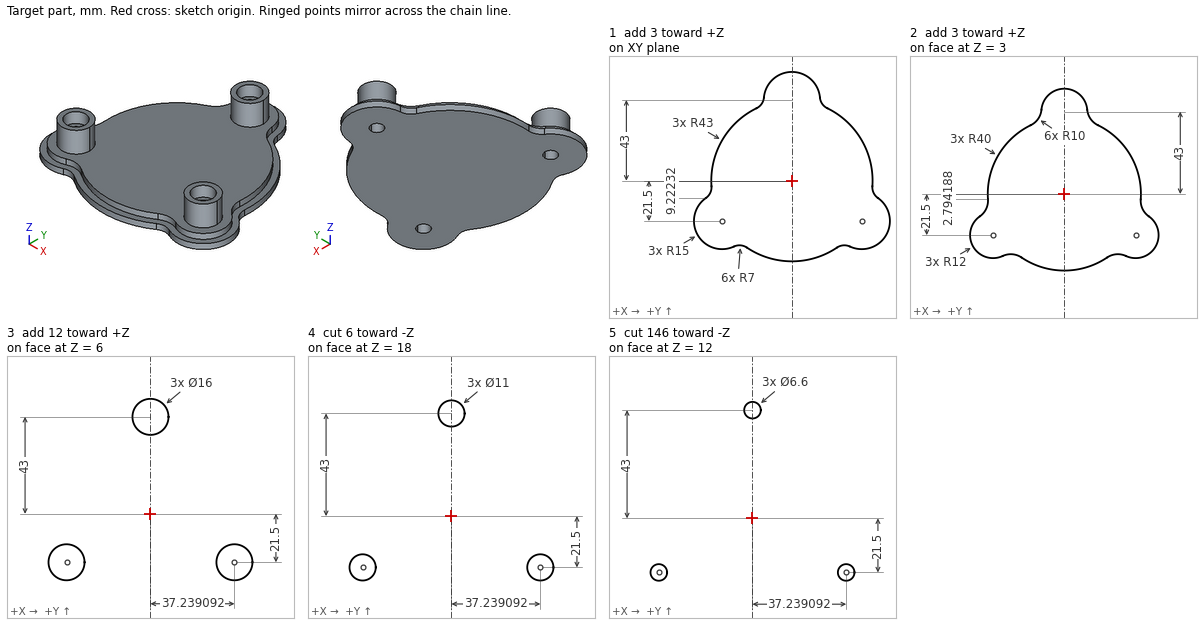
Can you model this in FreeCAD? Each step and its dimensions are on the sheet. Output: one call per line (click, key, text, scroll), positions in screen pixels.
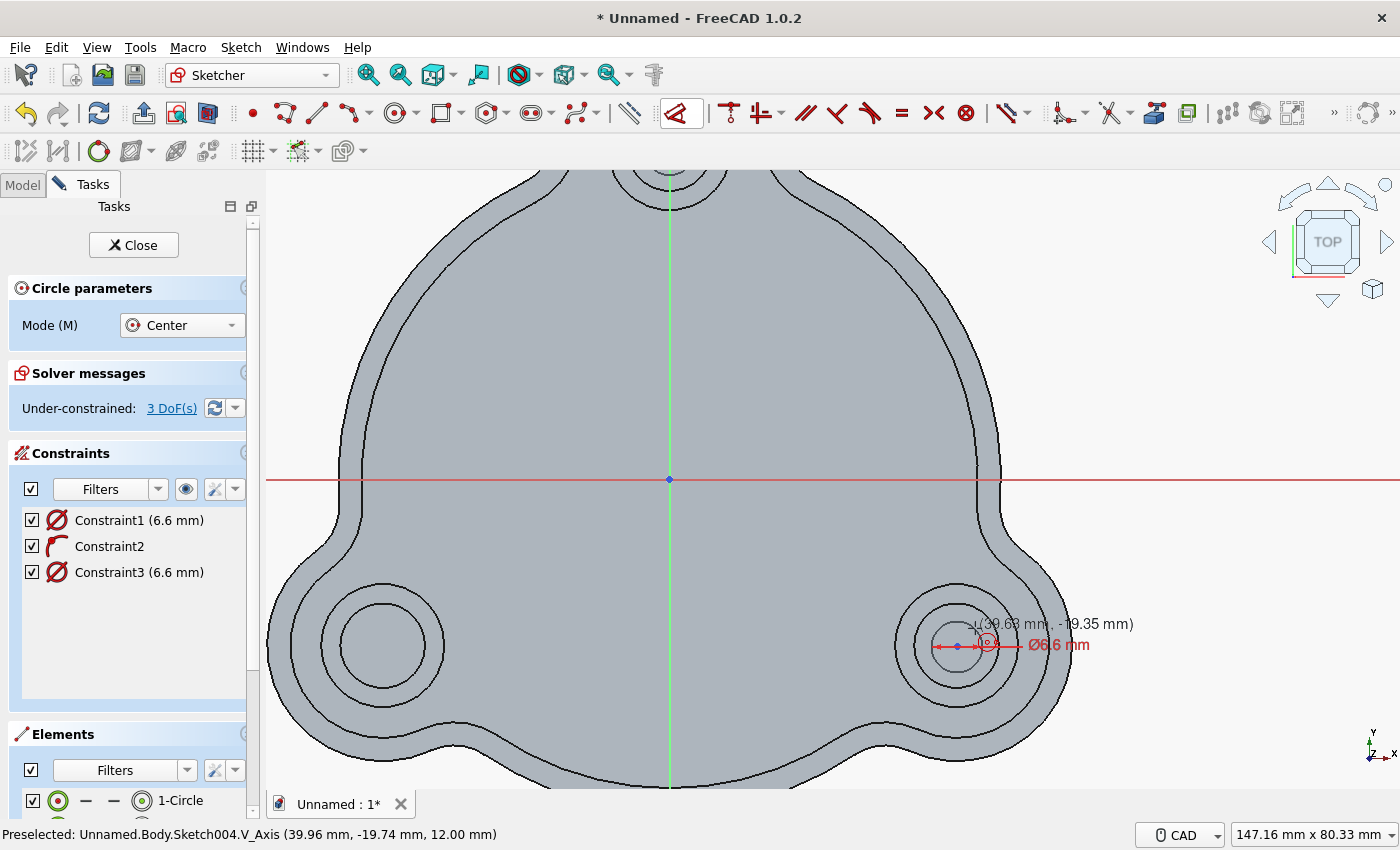
click(383, 646)
move(401, 628)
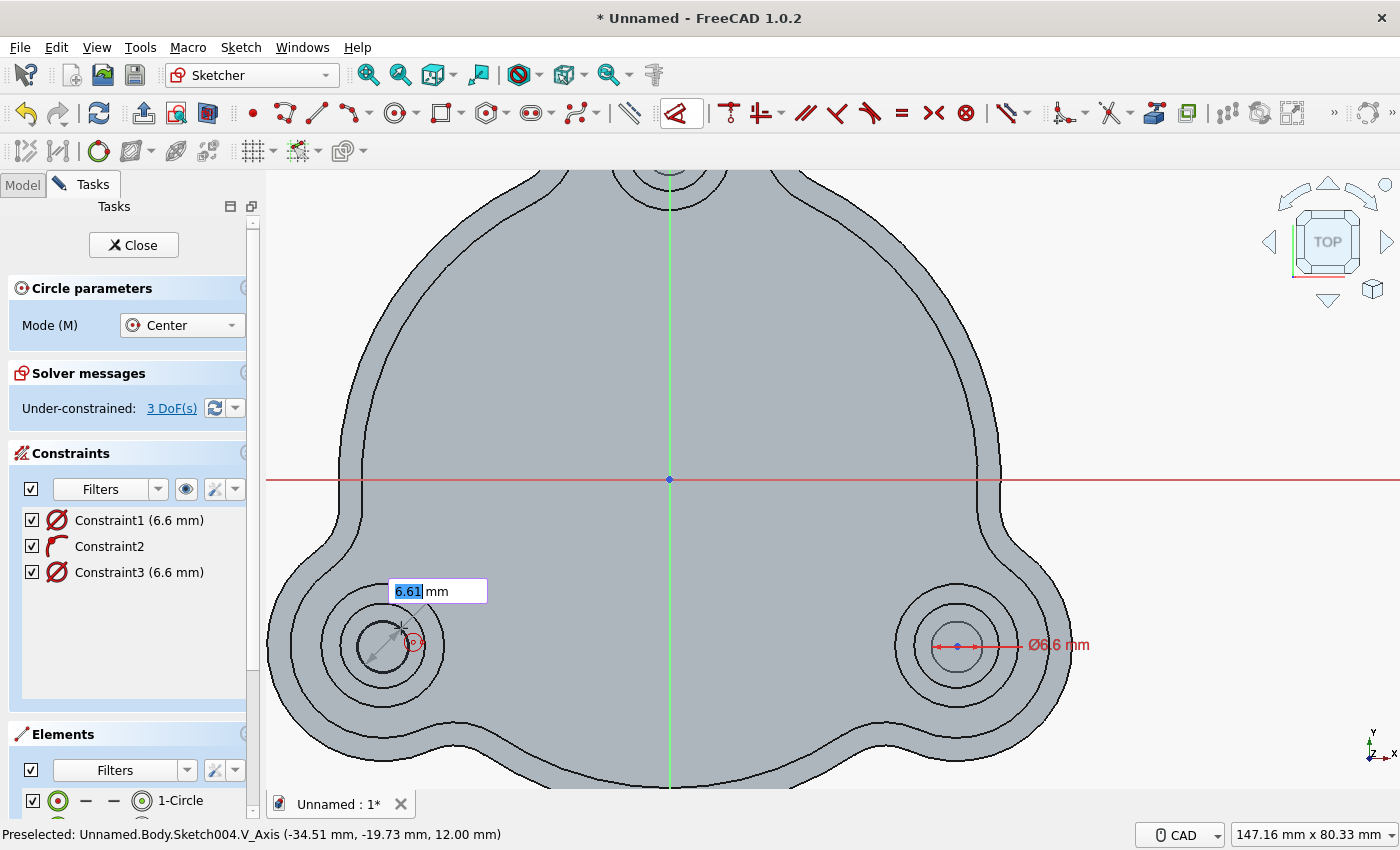
text(6.6)
key(Return)
key(Escape)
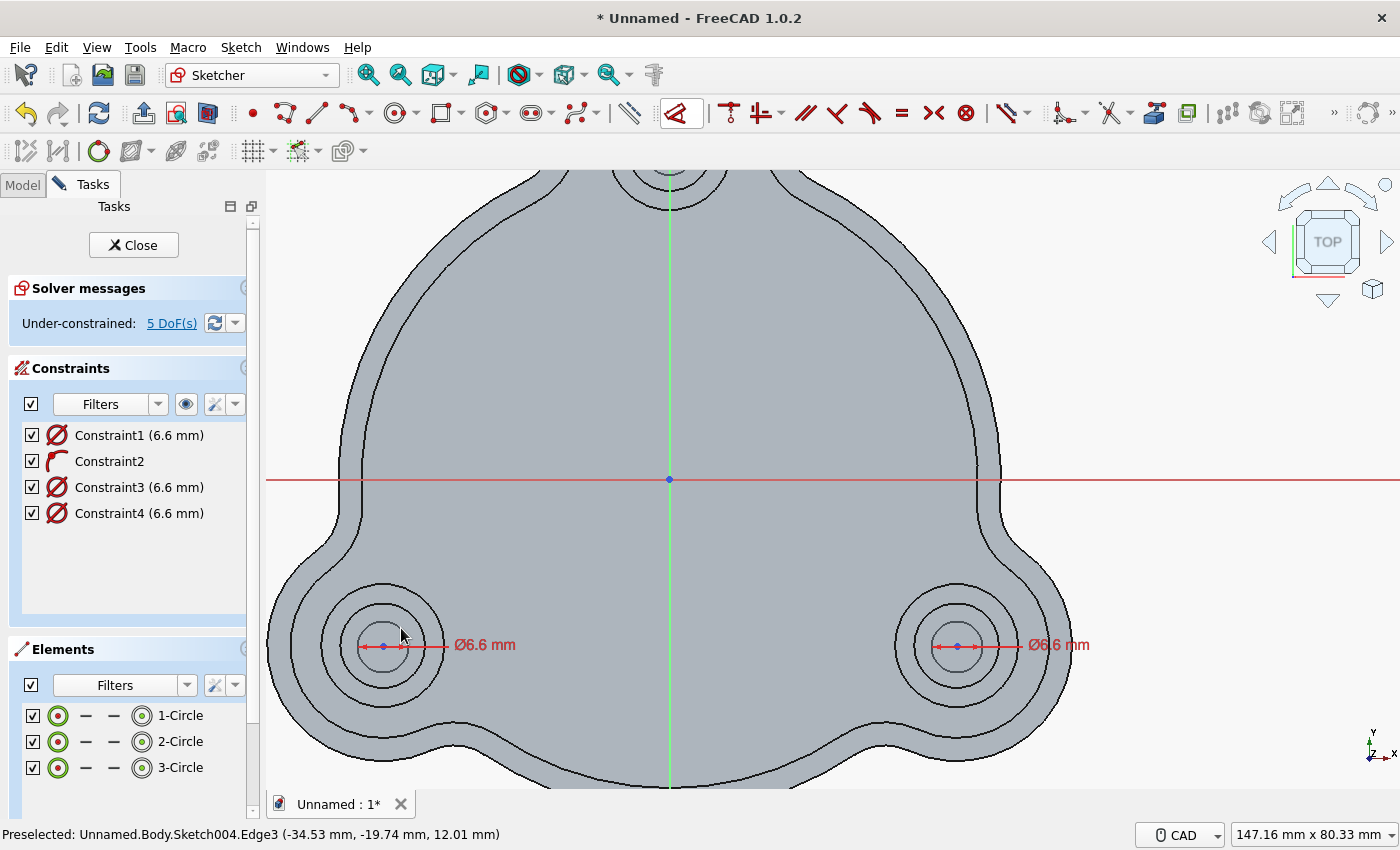
click(957, 647)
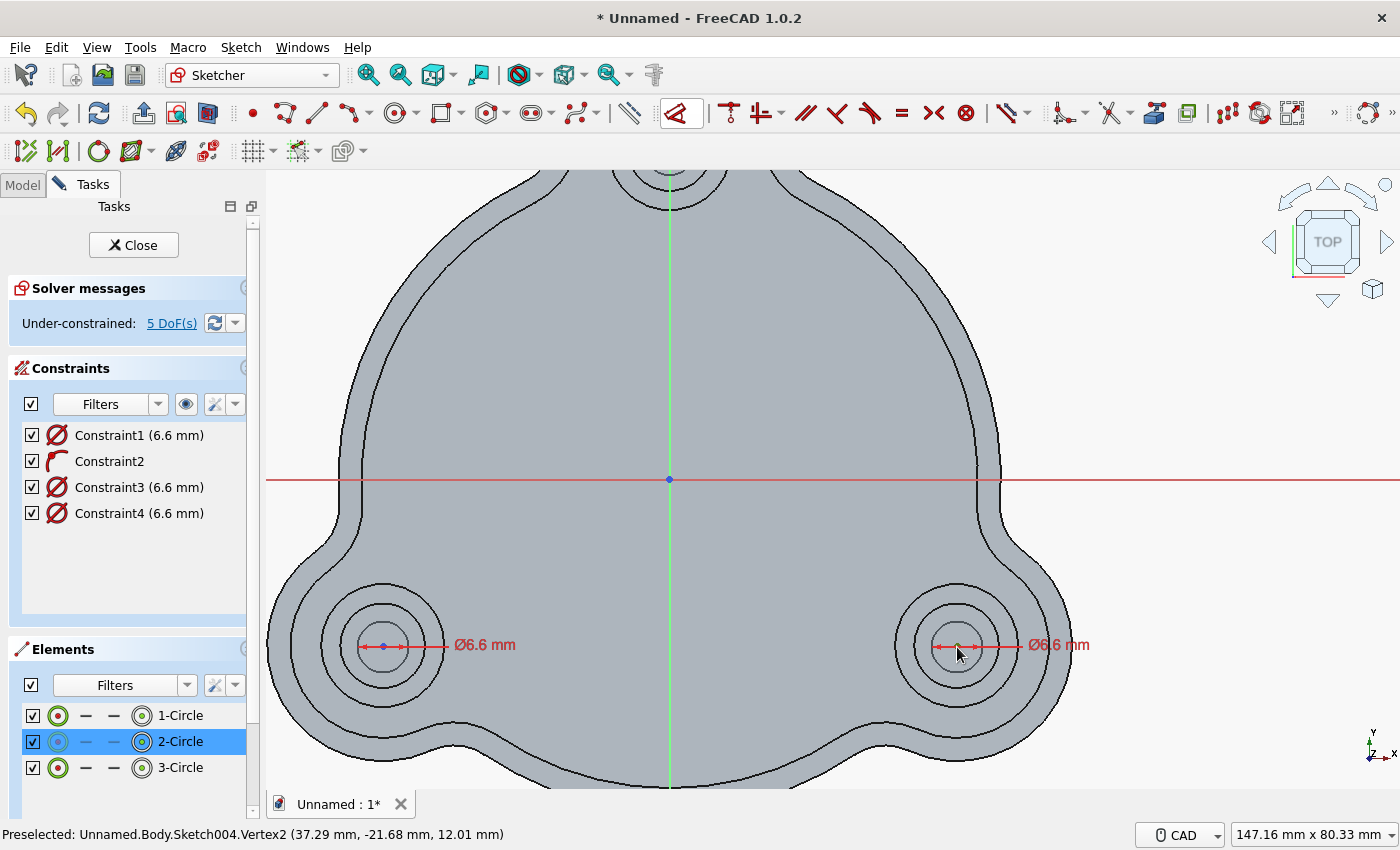
click(383, 647)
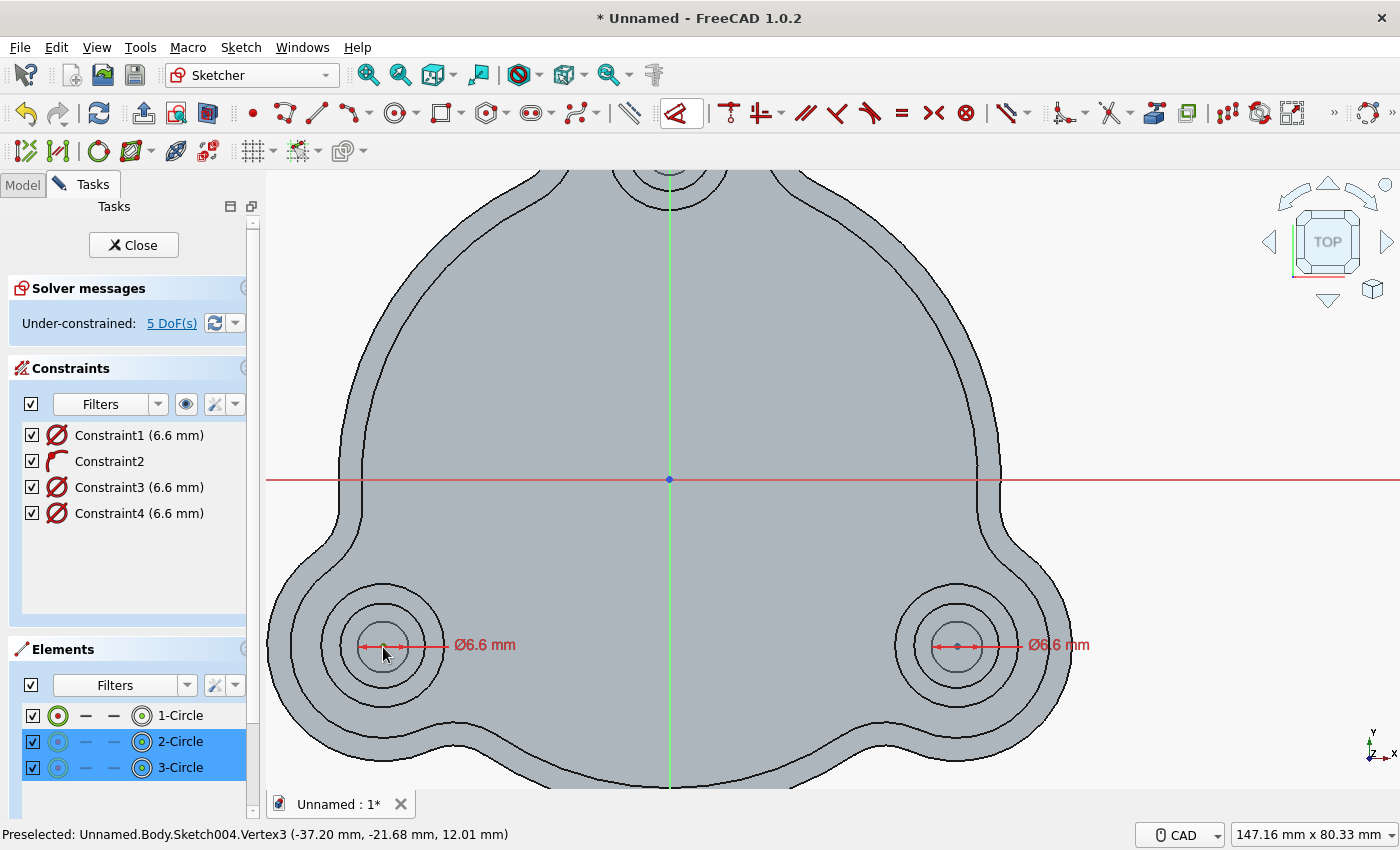
click(670, 721)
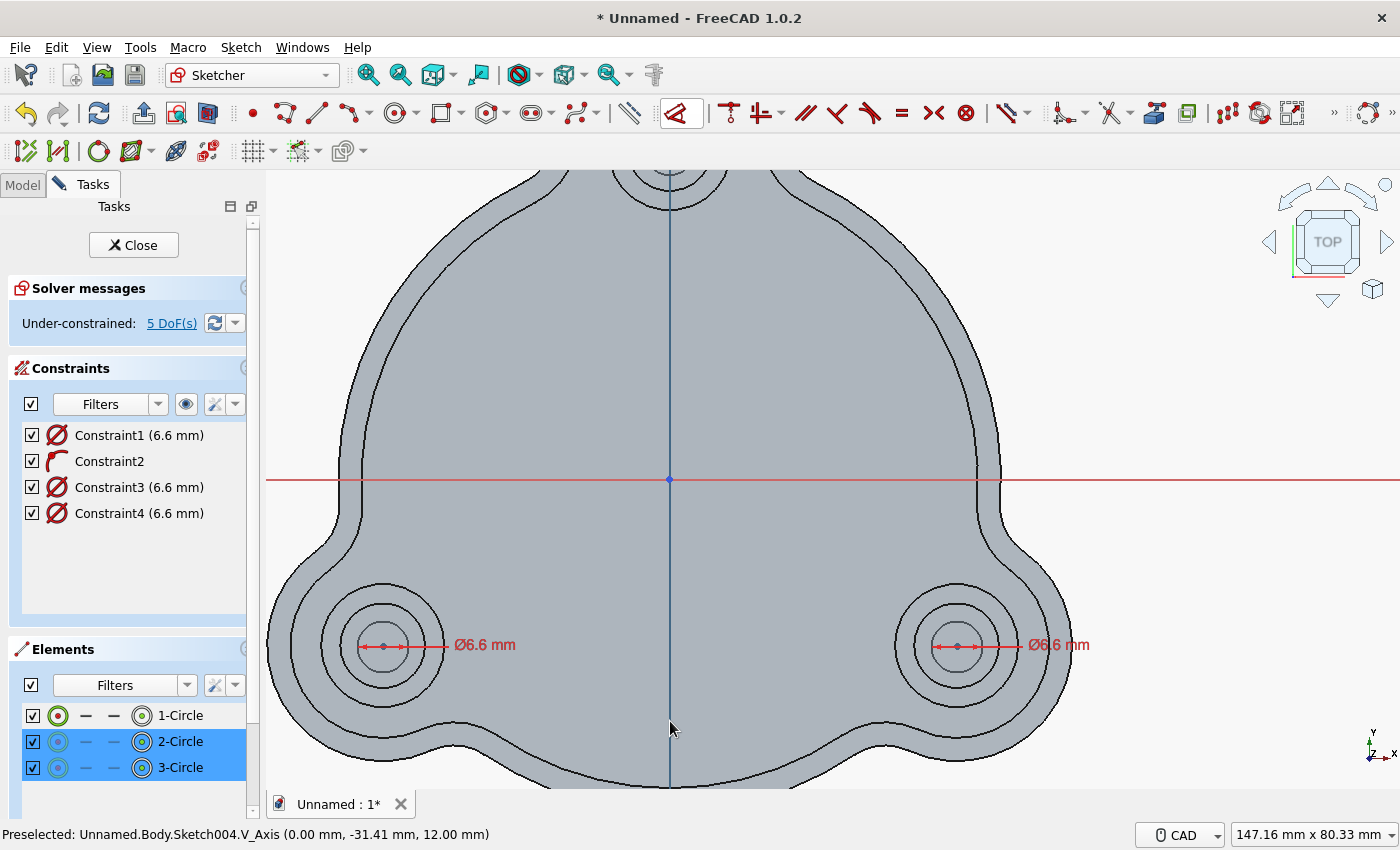
click(934, 114)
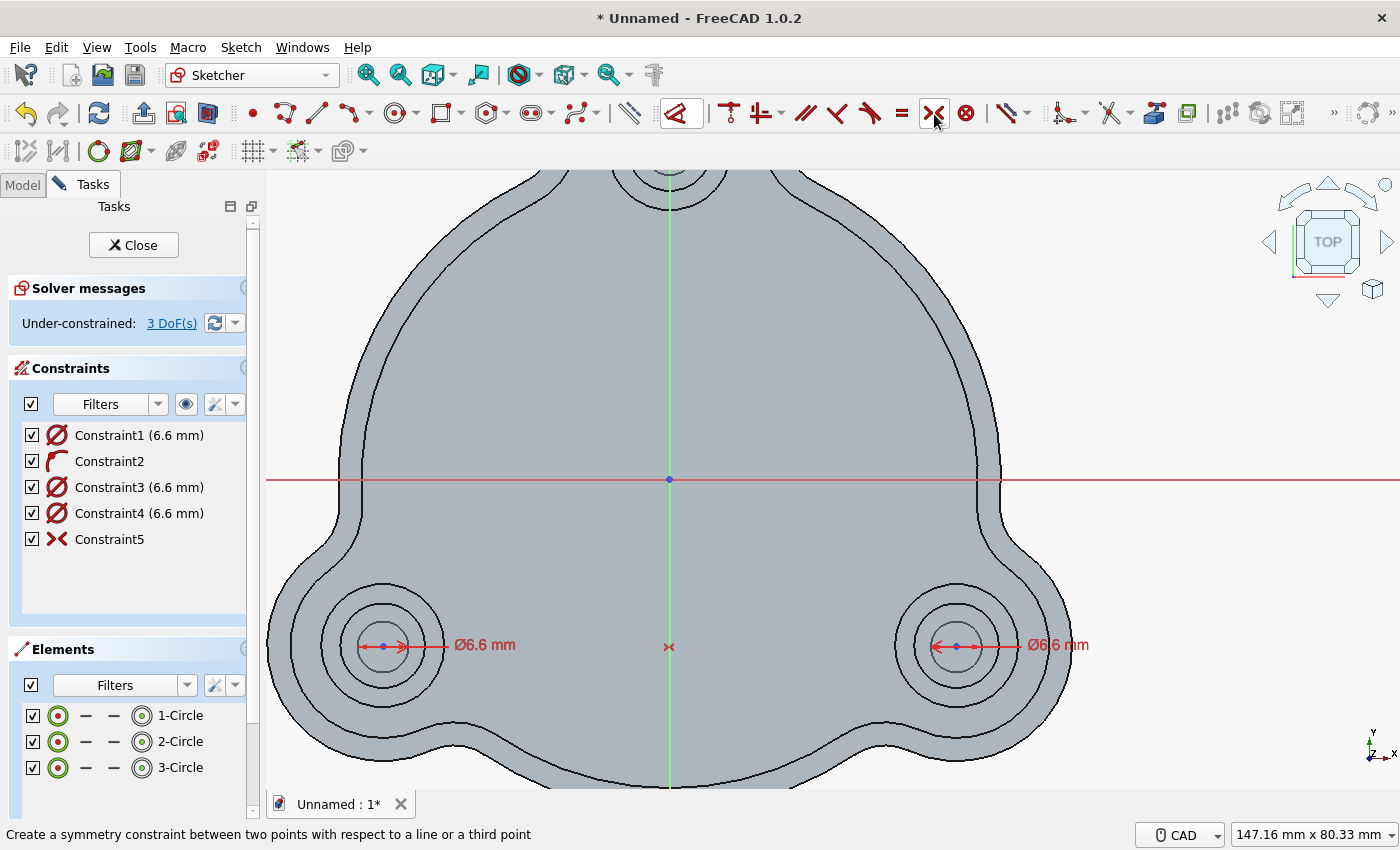
scroll(957, 647, down, 2)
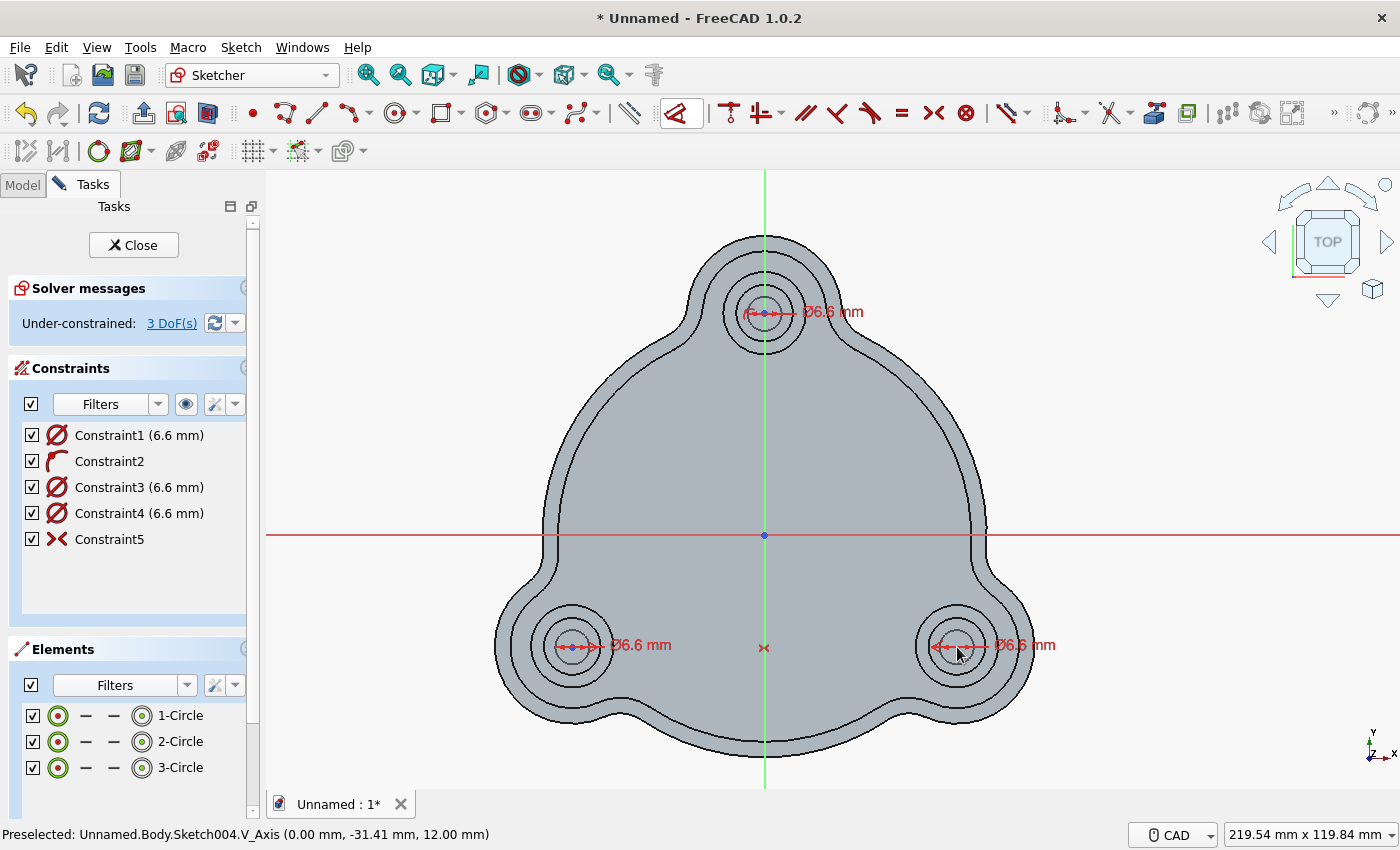
click(765, 314)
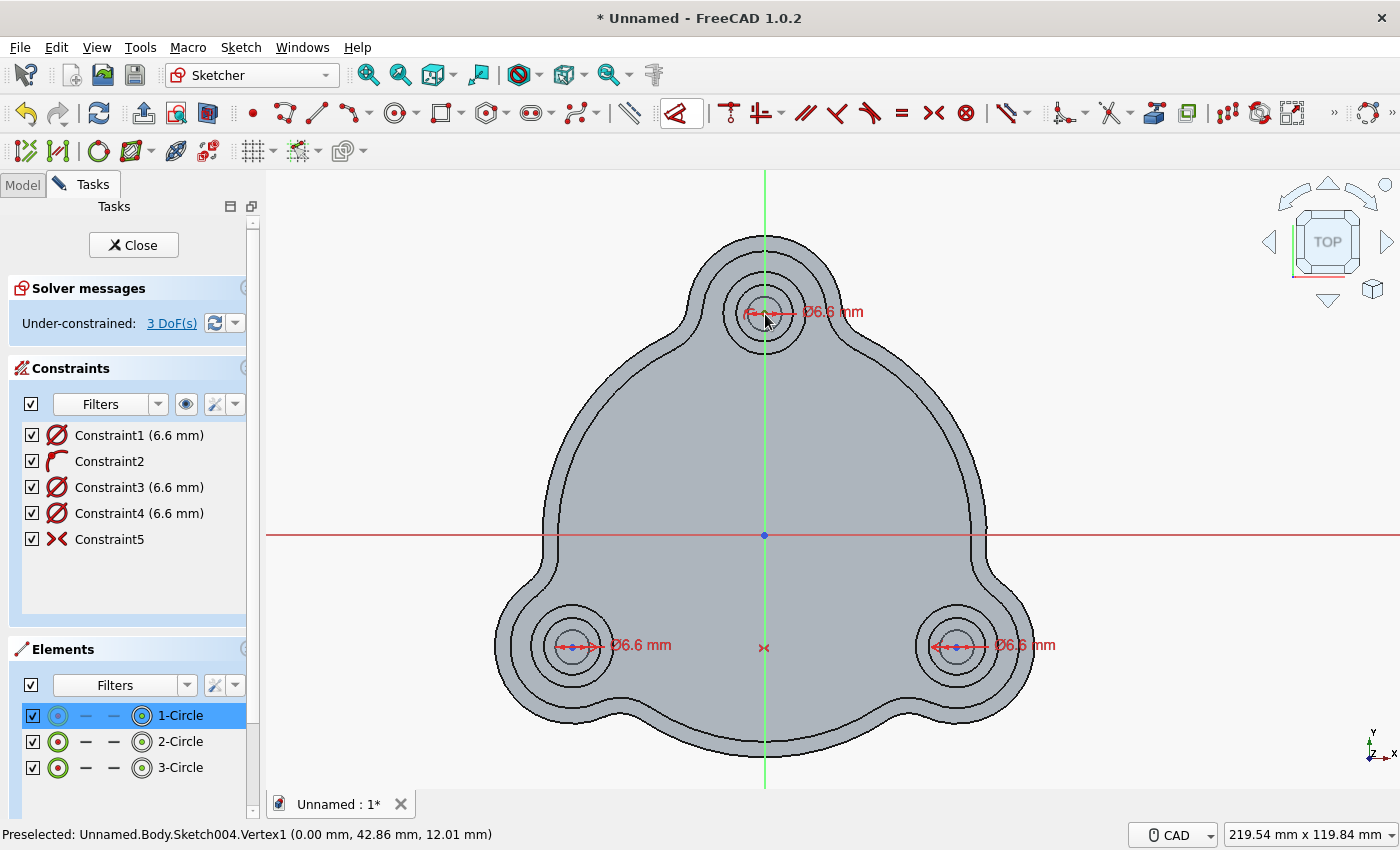
click(698, 114)